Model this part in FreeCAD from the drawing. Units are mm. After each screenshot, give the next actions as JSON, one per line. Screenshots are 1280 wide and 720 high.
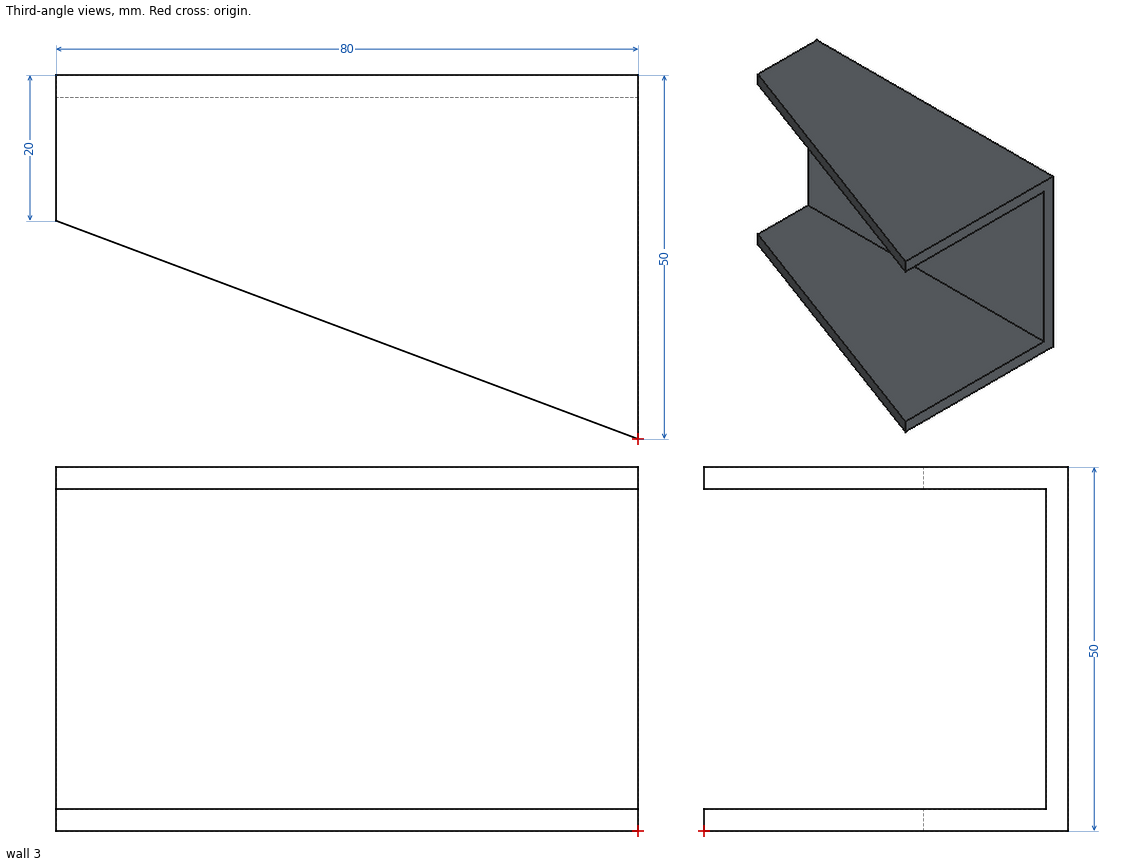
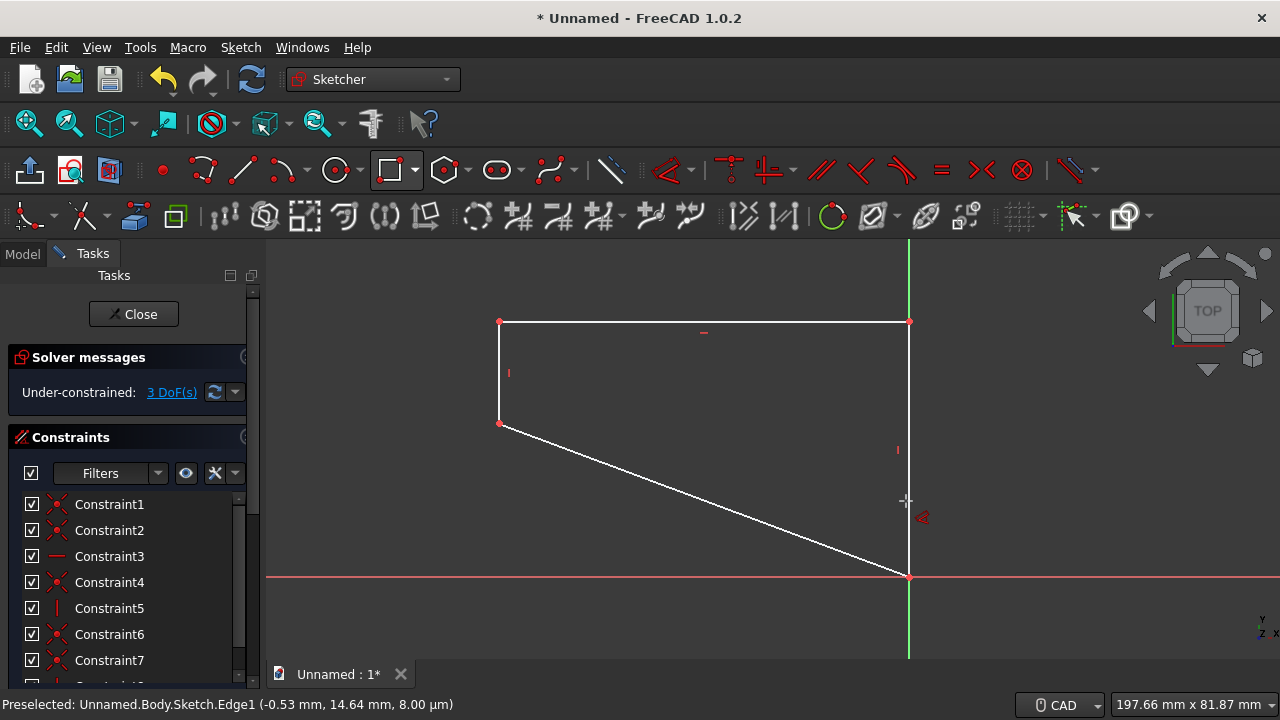
{"action": "left_click", "coordinate": [909, 501]}
{"action": "left_click", "coordinate": [943, 450]}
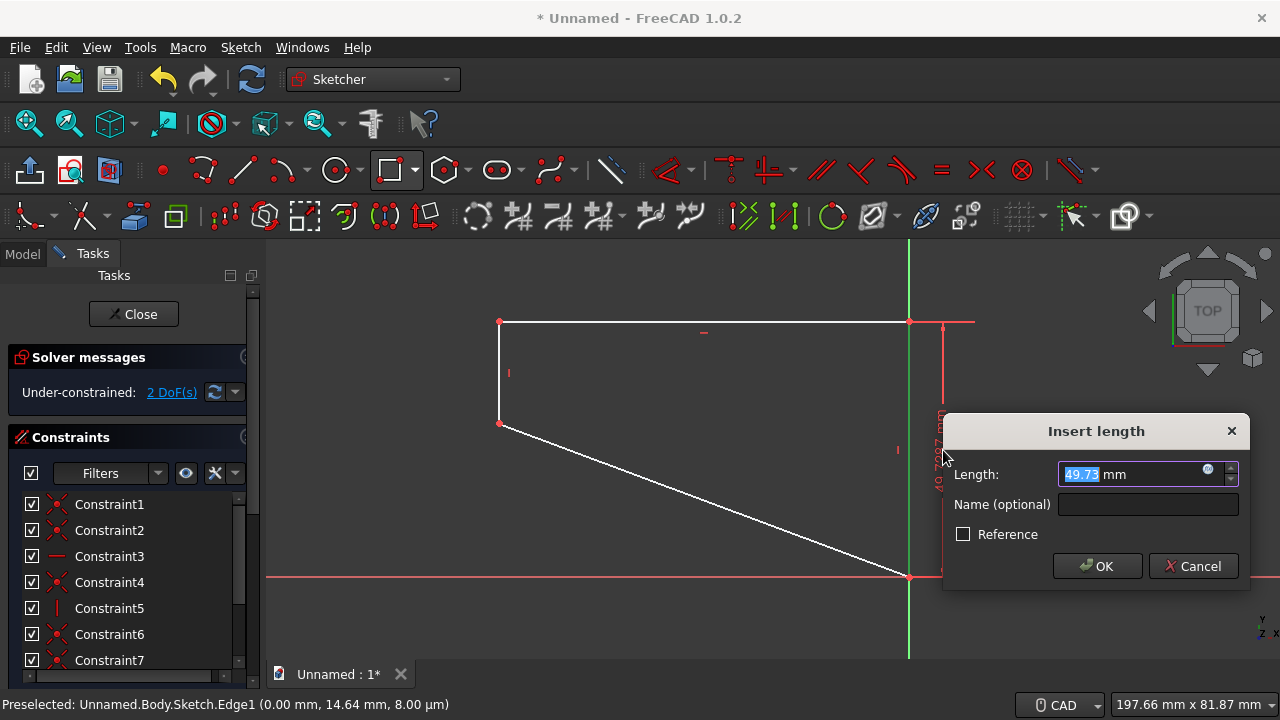
{"action": "type", "text": "50"}
{"action": "key", "text": "Return"}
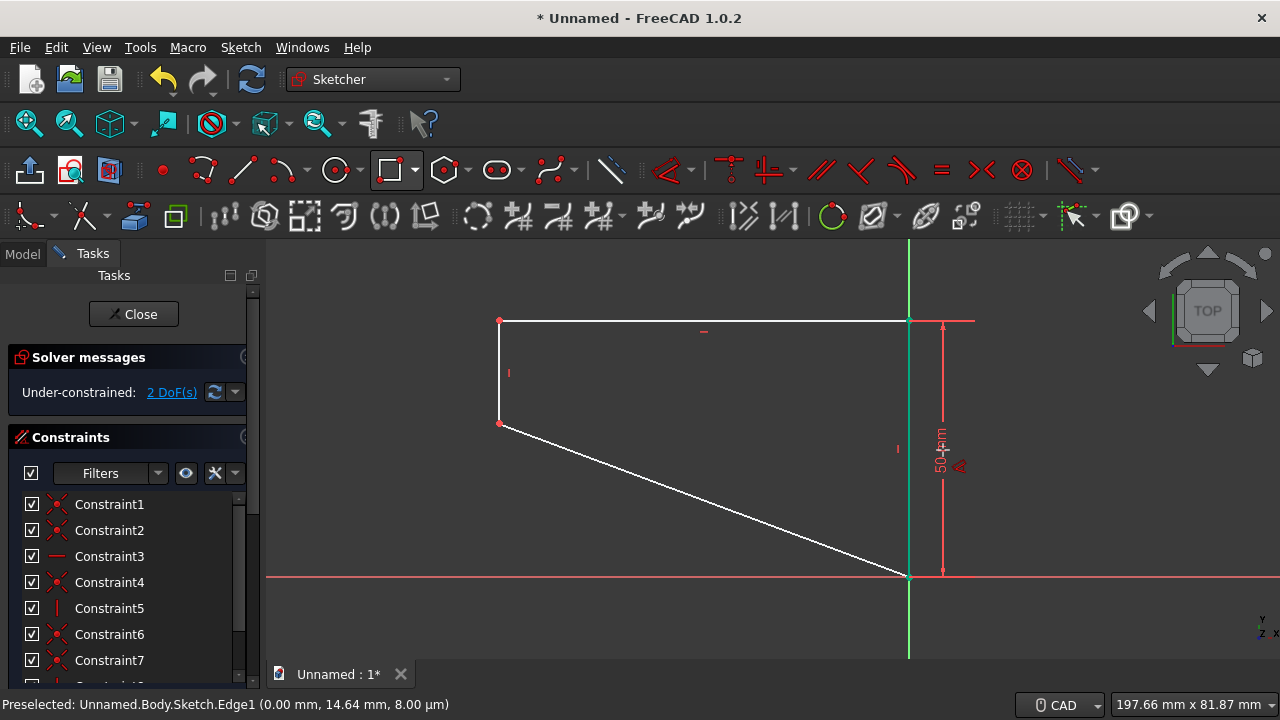
{"action": "left_click", "coordinate": [786, 321]}
{"action": "left_click", "coordinate": [704, 287]}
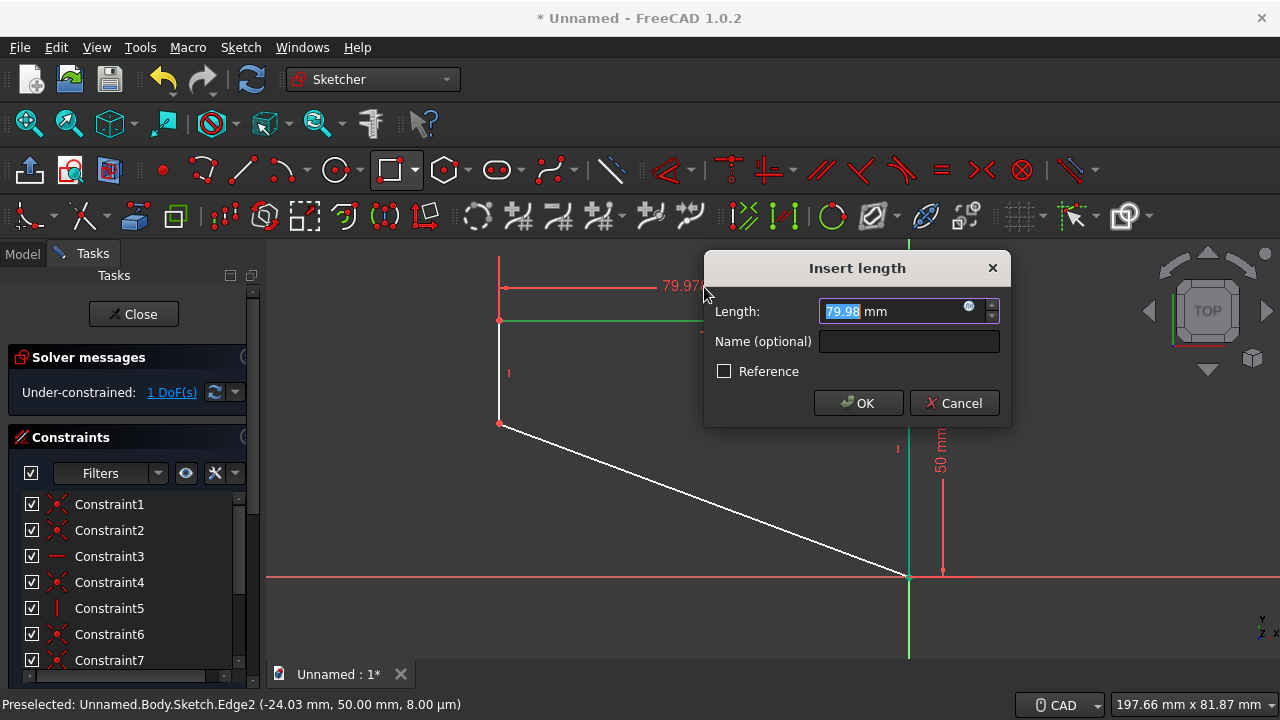
{"action": "type", "text": "80"}
{"action": "key", "text": "Return"}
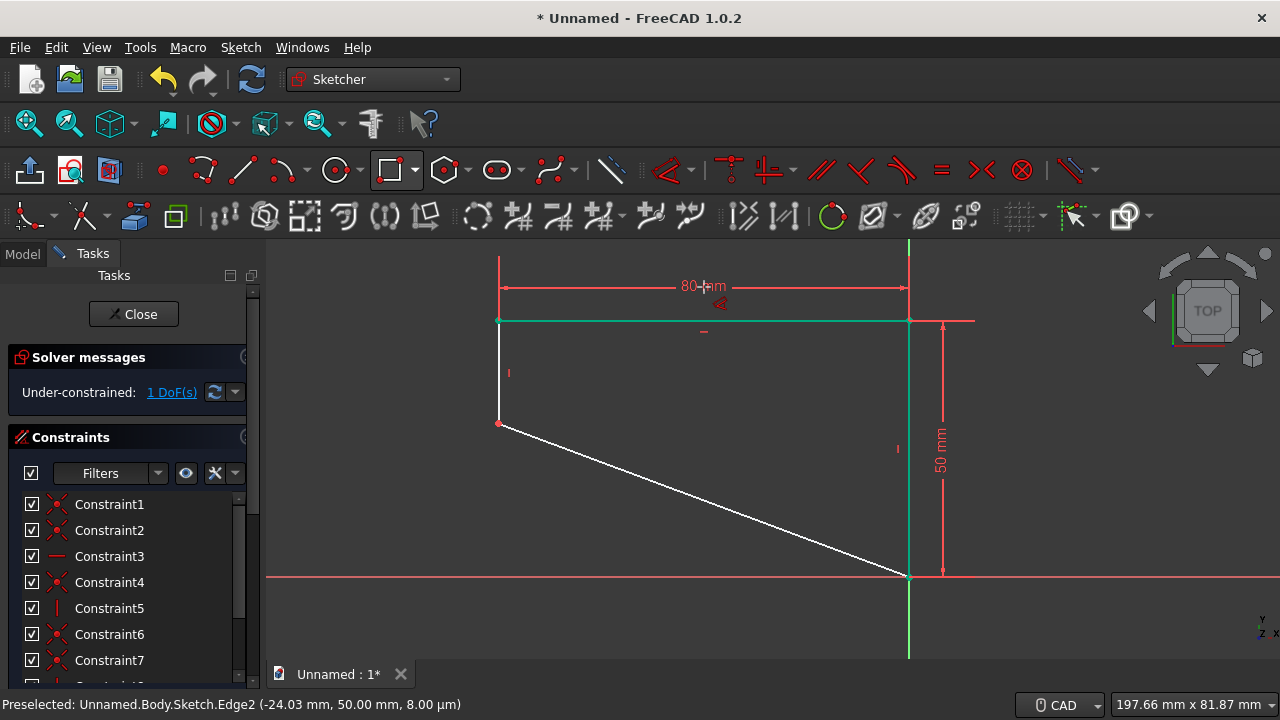
{"action": "left_click", "coordinate": [499, 352]}
{"action": "left_click", "coordinate": [465, 372]}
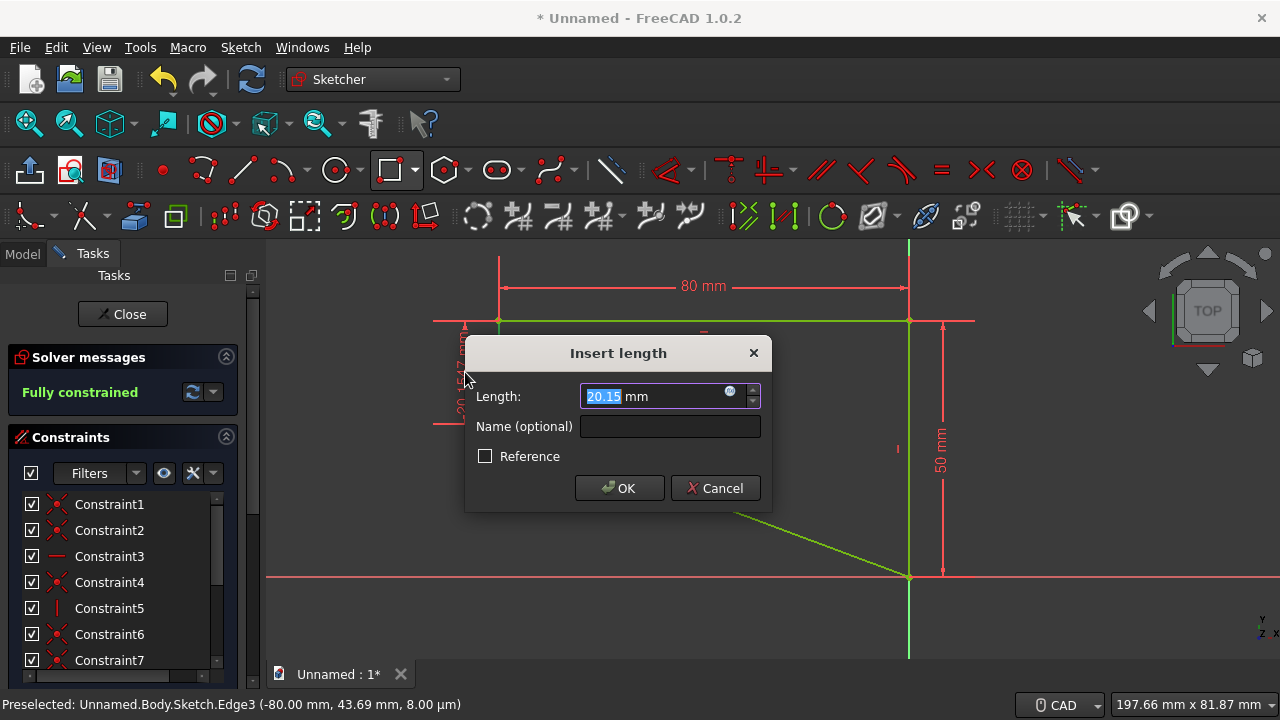
{"action": "type", "text": "20"}
{"action": "key", "text": "Return"}
{"action": "key", "text": "Escape"}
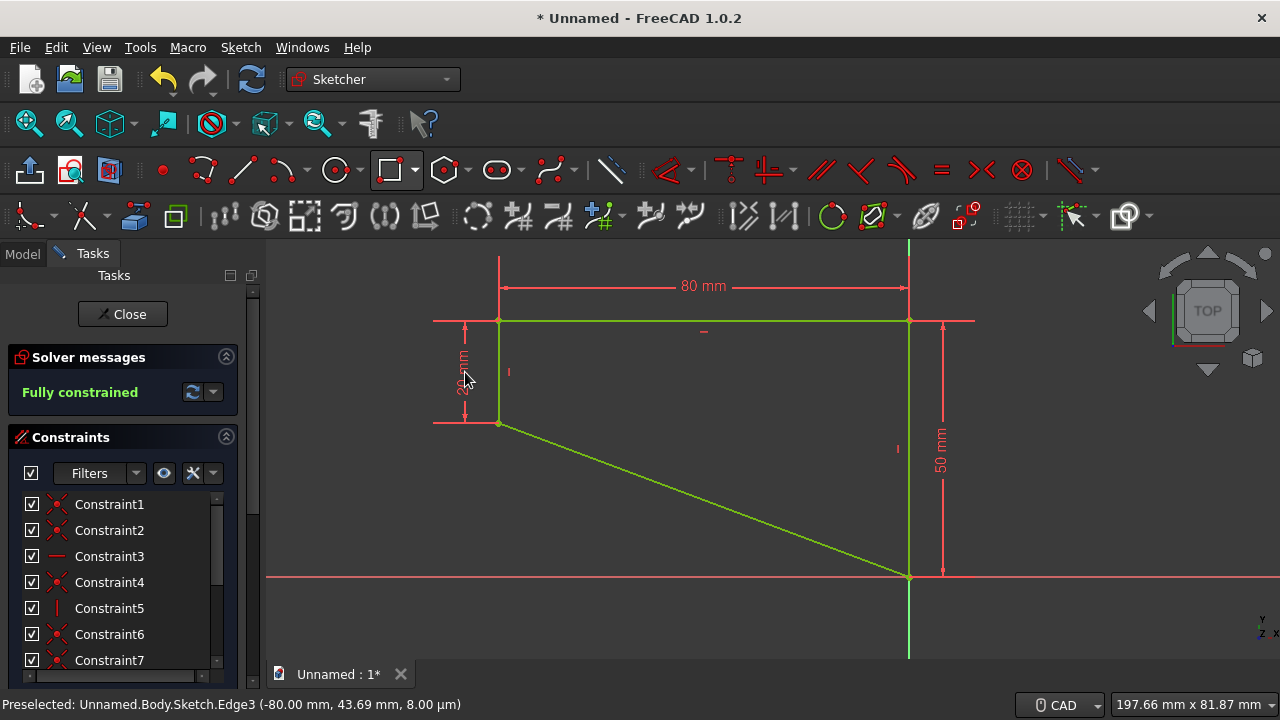
{"action": "left_click", "coordinate": [123, 314]}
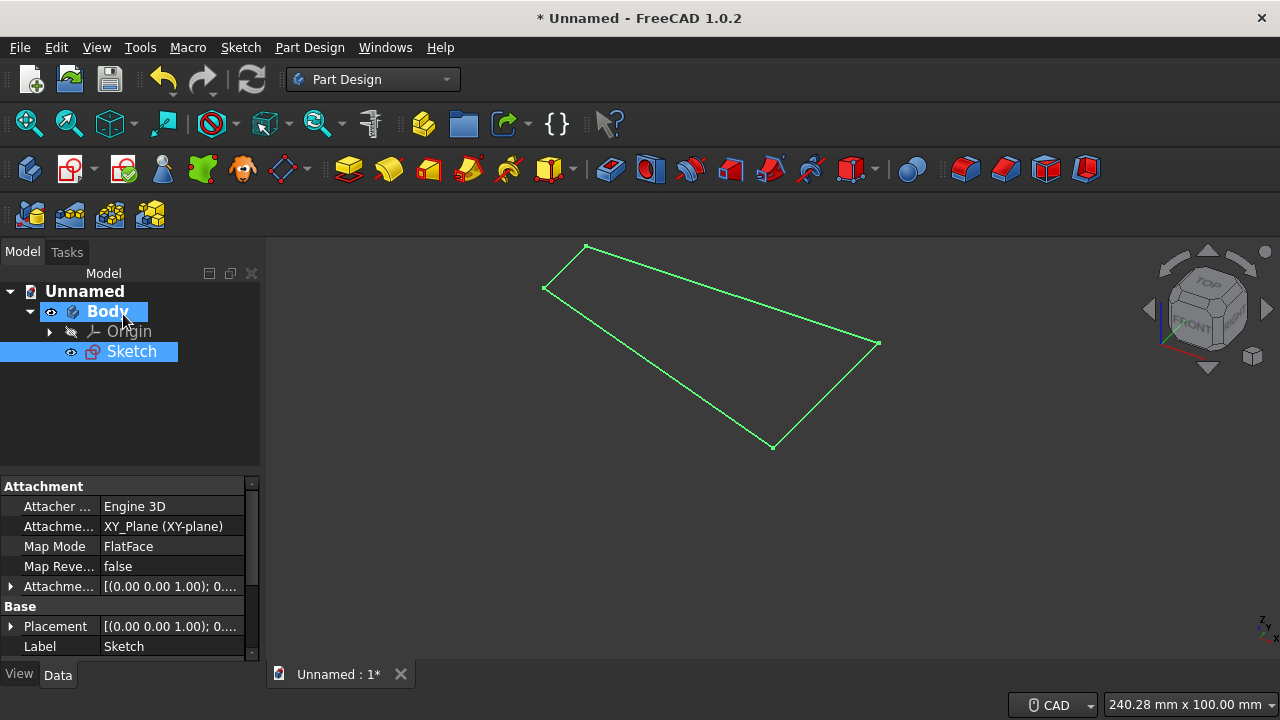
{"action": "left_click", "coordinate": [350, 170]}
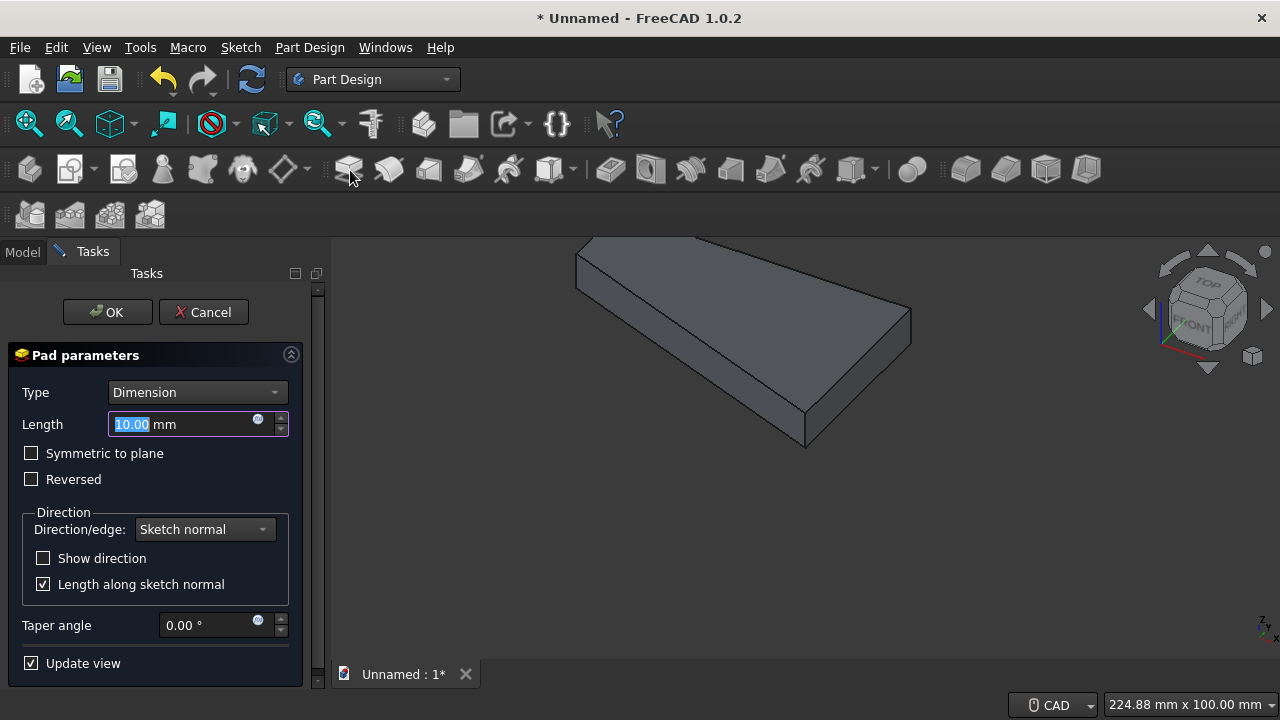
{"action": "type", "text": "50"}
{"action": "key", "text": "Tab"}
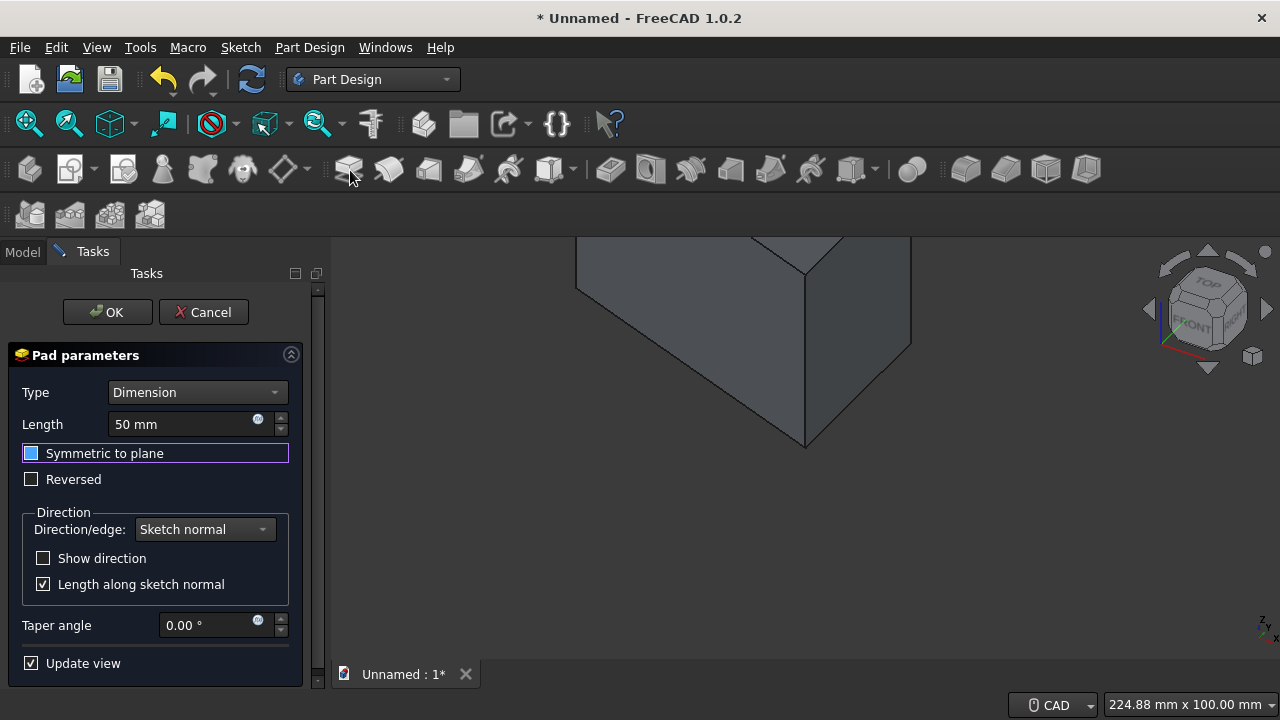
{"action": "left_click", "coordinate": [108, 312]}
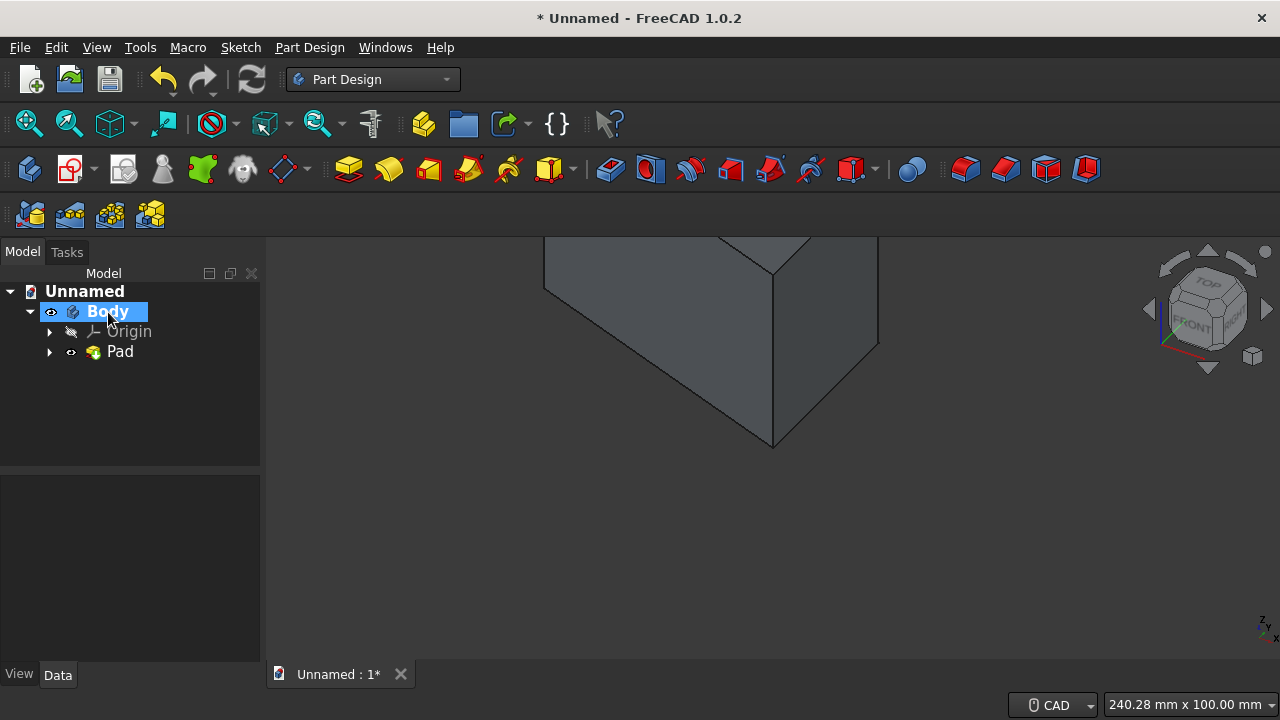
{"action": "key", "text": "v f"}